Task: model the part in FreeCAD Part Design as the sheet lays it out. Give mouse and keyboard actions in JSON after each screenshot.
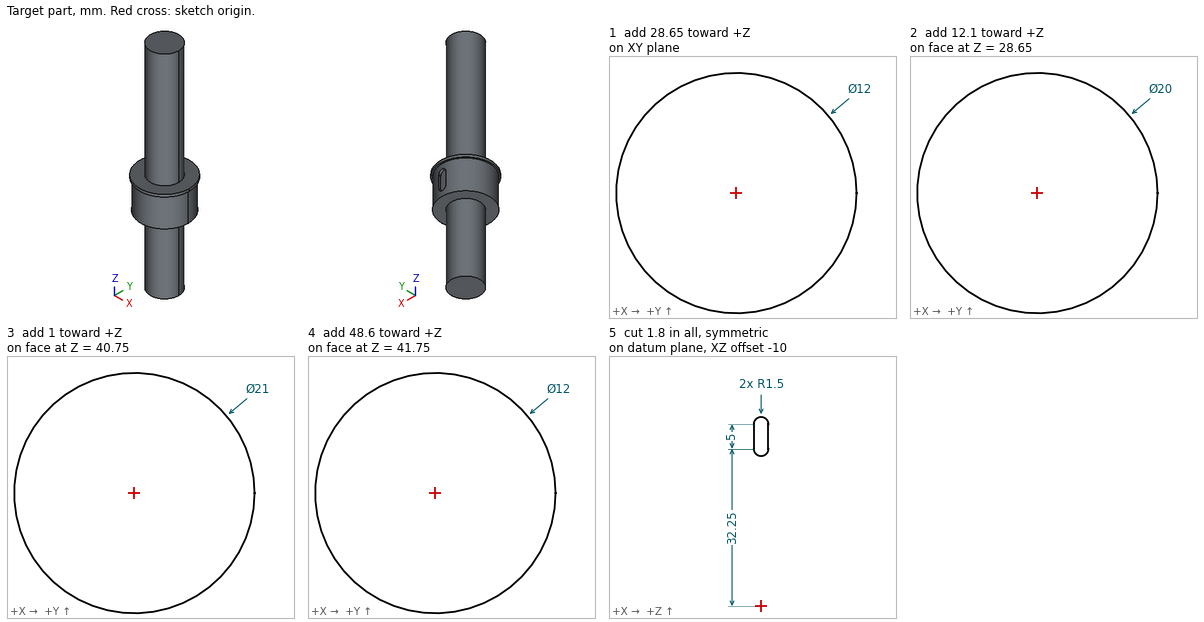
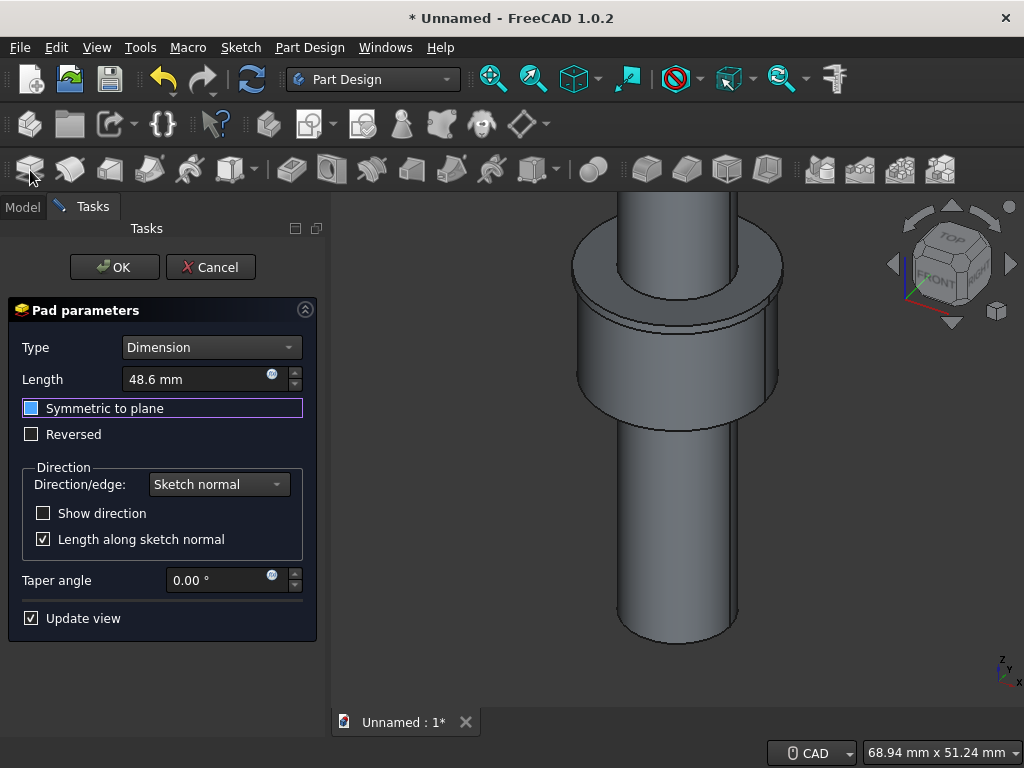
{"action": "left_click", "coordinate": [115, 267]}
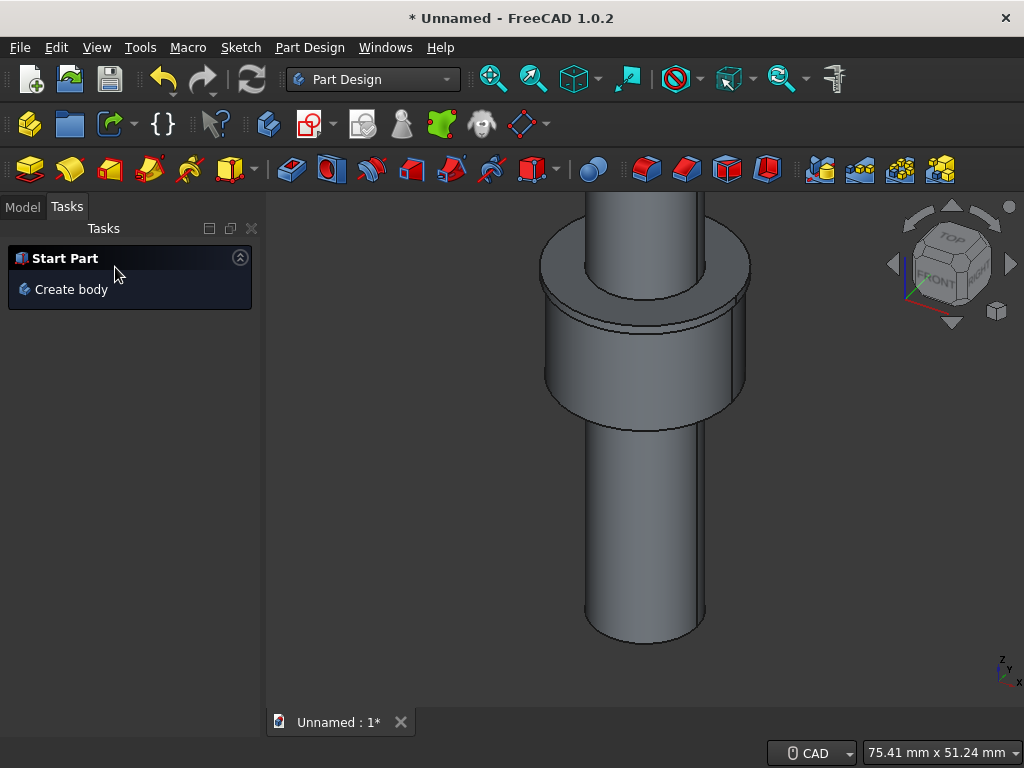
{"action": "left_click", "coordinate": [494, 80]}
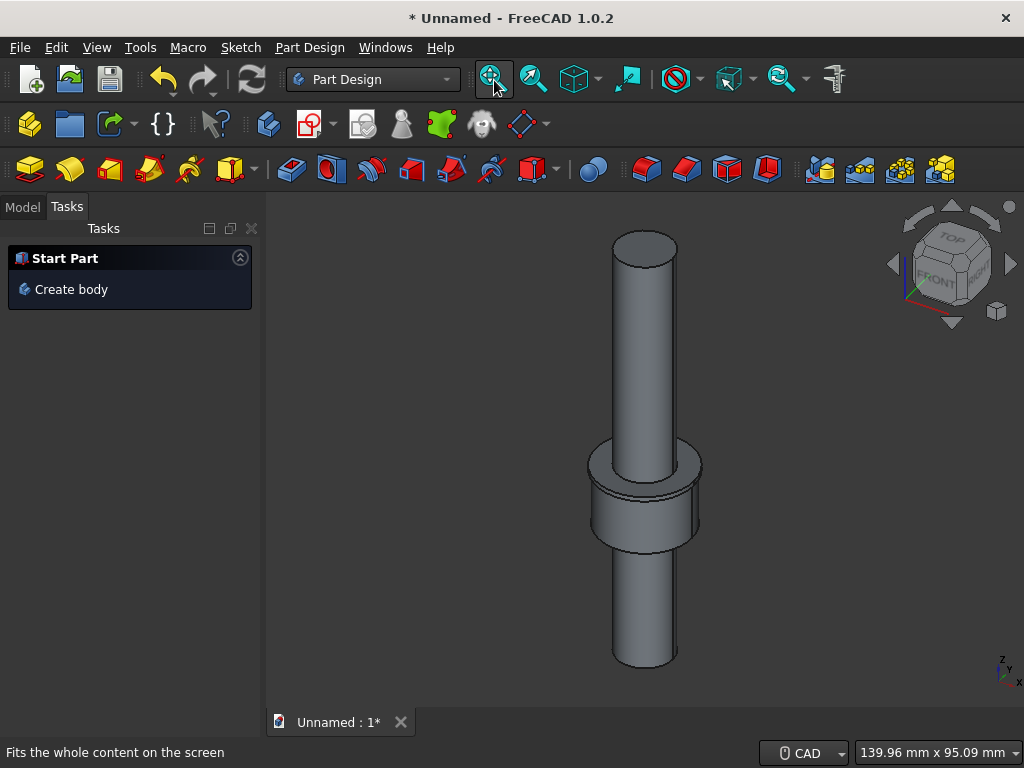
{"action": "left_click", "coordinate": [23, 206]}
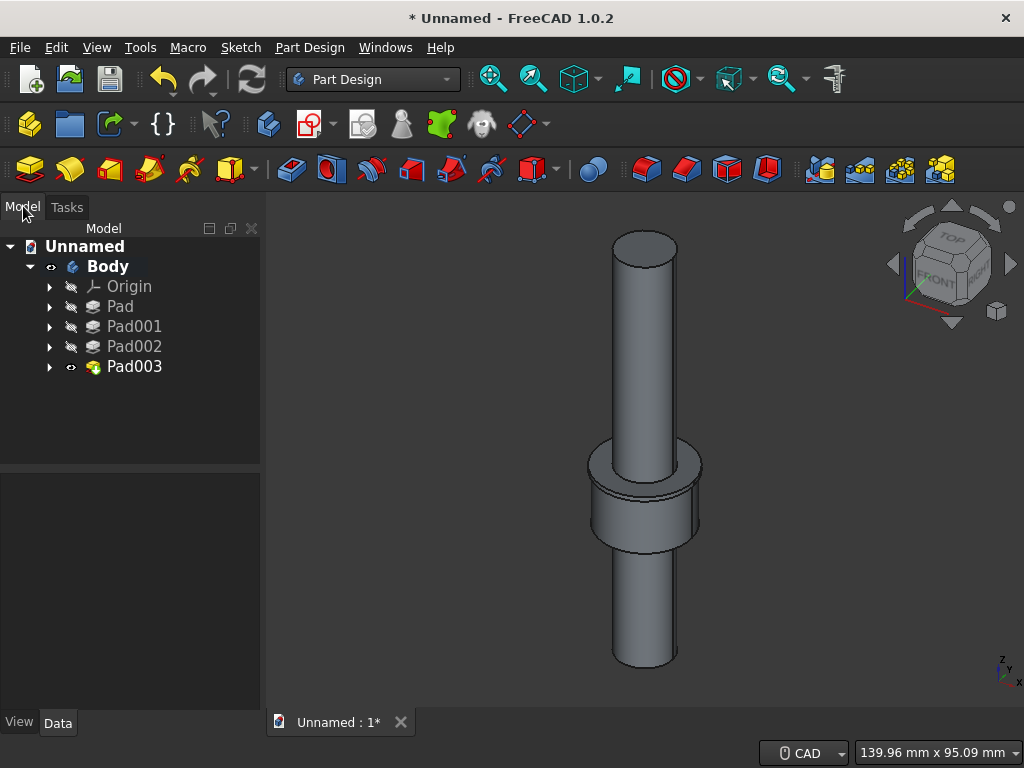
{"action": "left_click", "coordinate": [50, 287]}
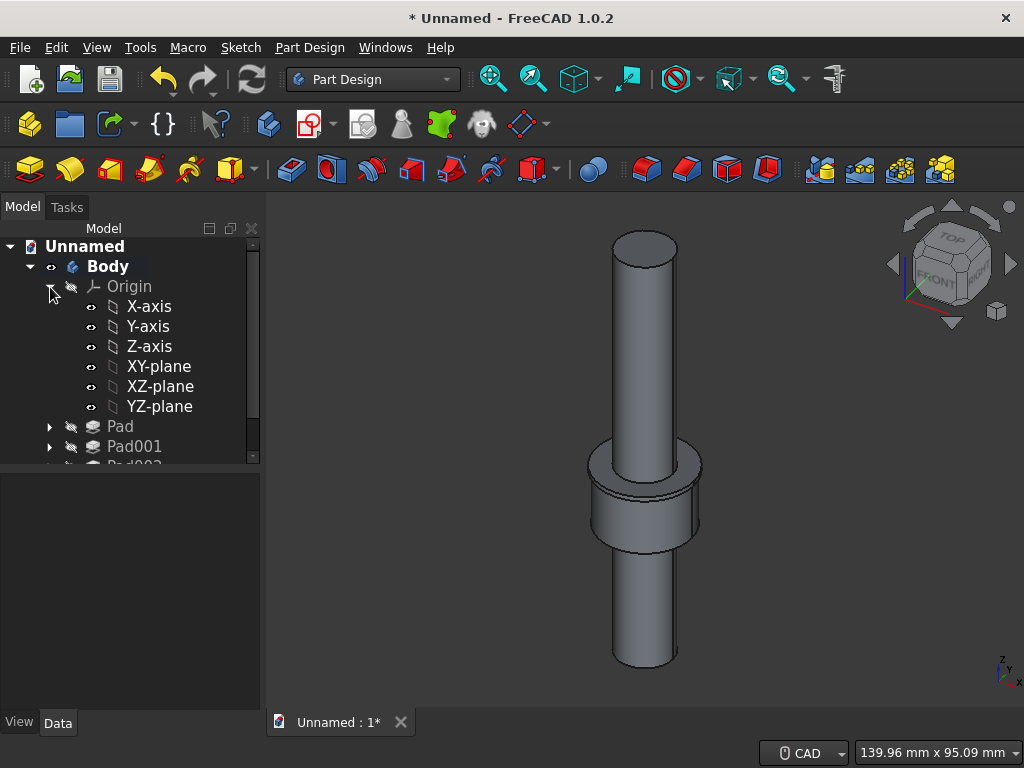
{"action": "left_click", "coordinate": [136, 387]}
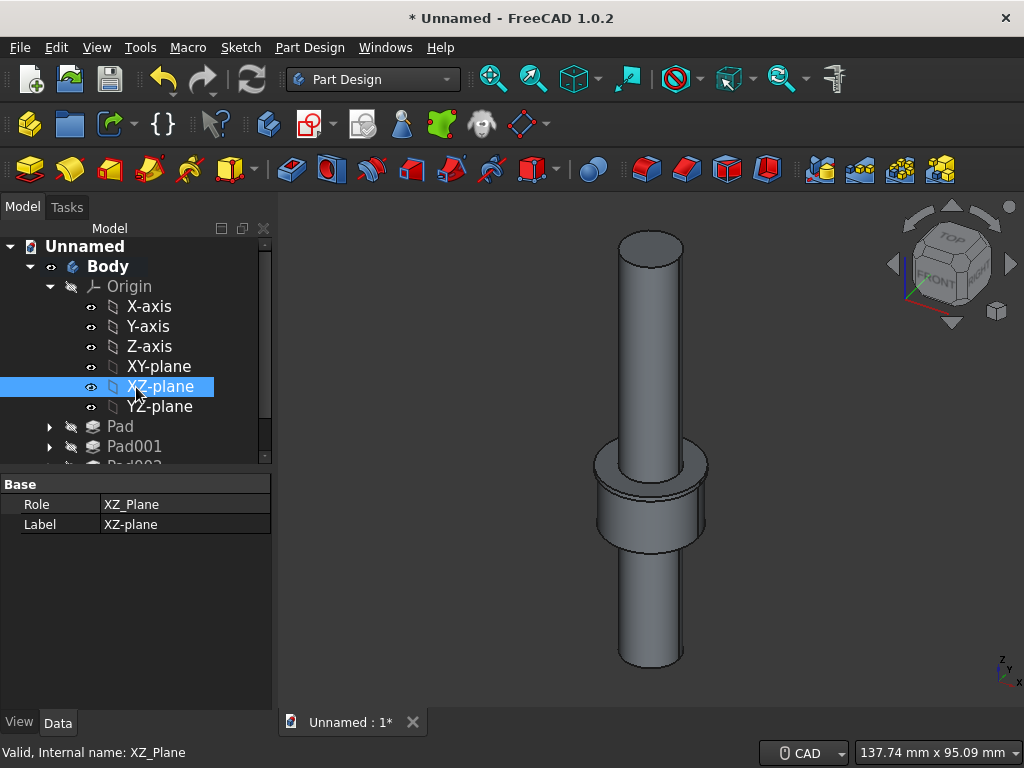
{"action": "left_click", "coordinate": [522, 124]}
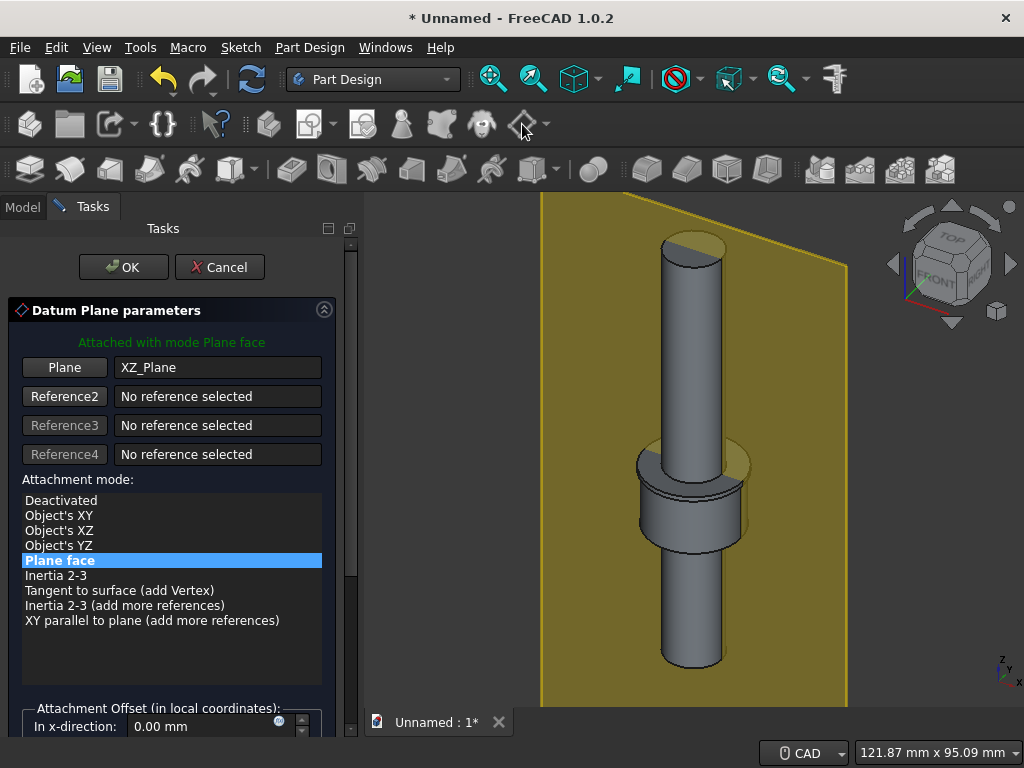
{"action": "scroll", "coordinate": [351, 487], "scroll_direction": "down", "scroll_amount": 3}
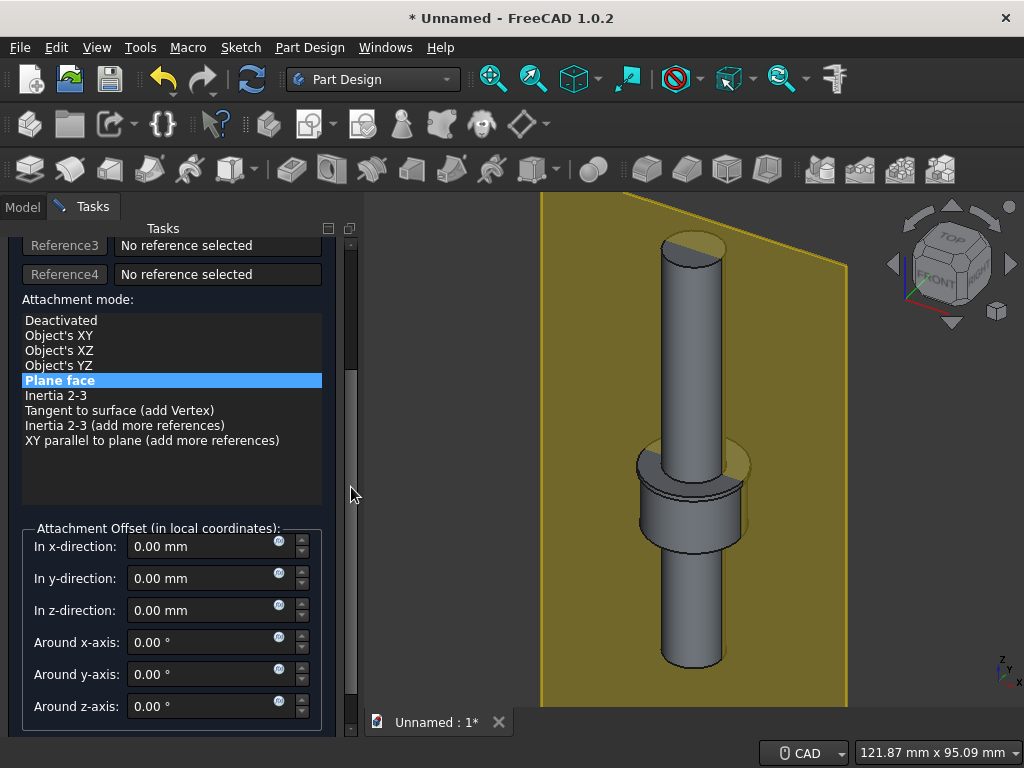
{"action": "triple_click", "coordinate": [210, 610]}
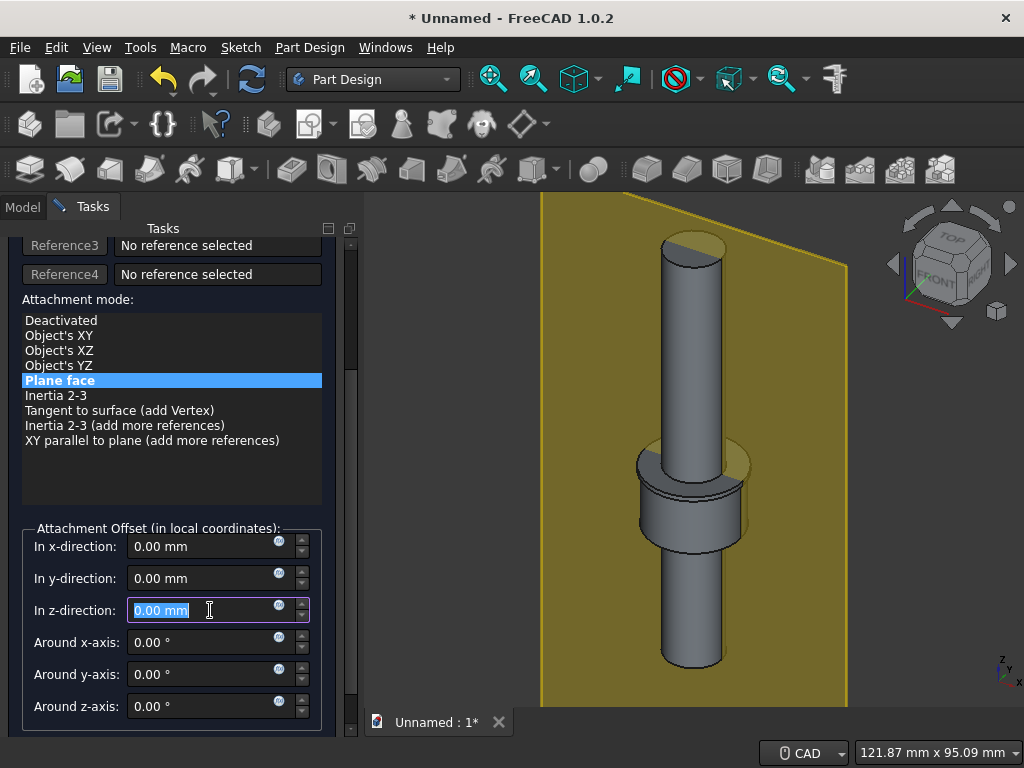
{"action": "type", "text": "-10"}
{"action": "key", "text": "Tab"}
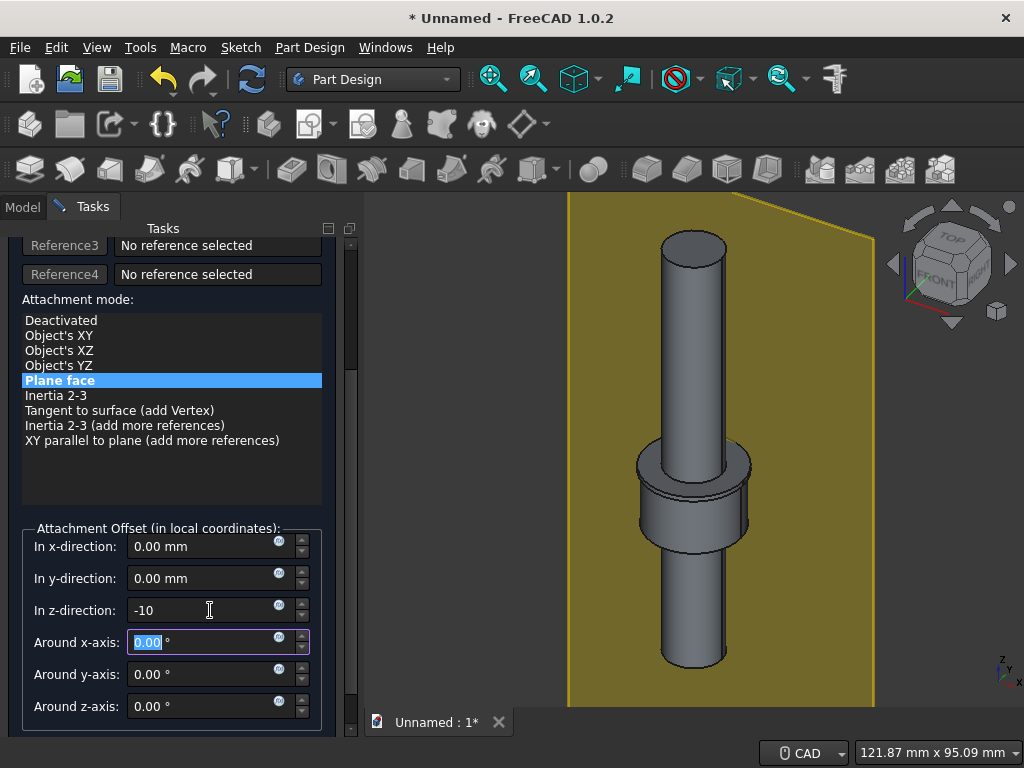
{"action": "scroll", "coordinate": [351, 487], "scroll_direction": "up", "scroll_amount": 4}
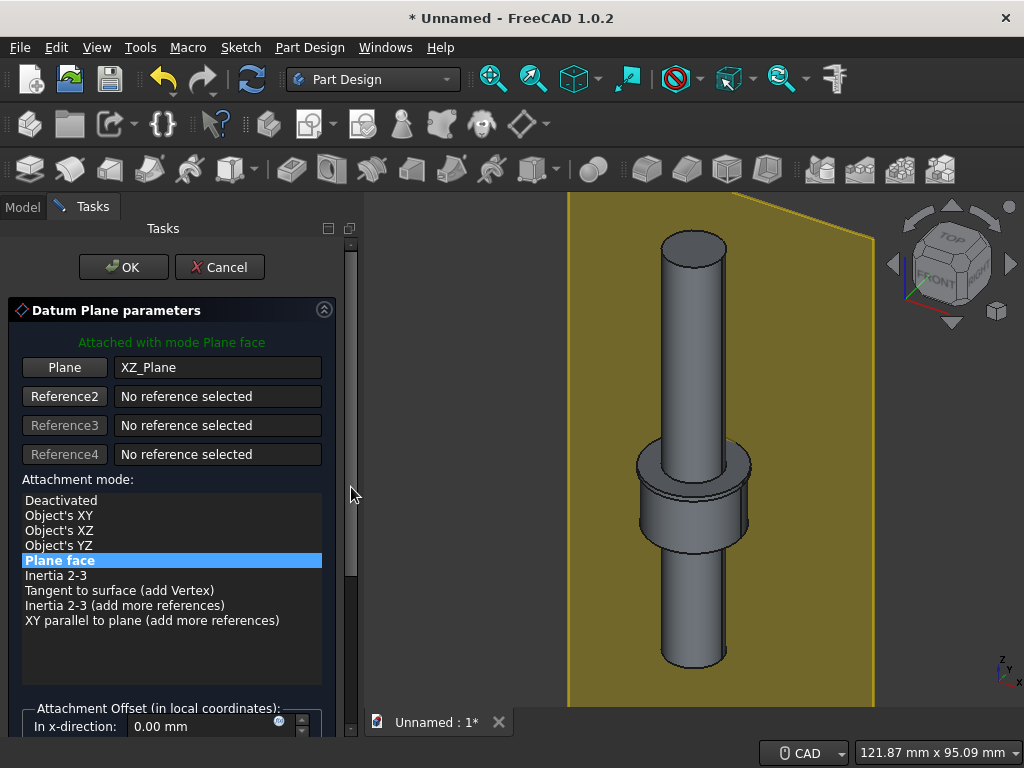
{"action": "left_click", "coordinate": [124, 267]}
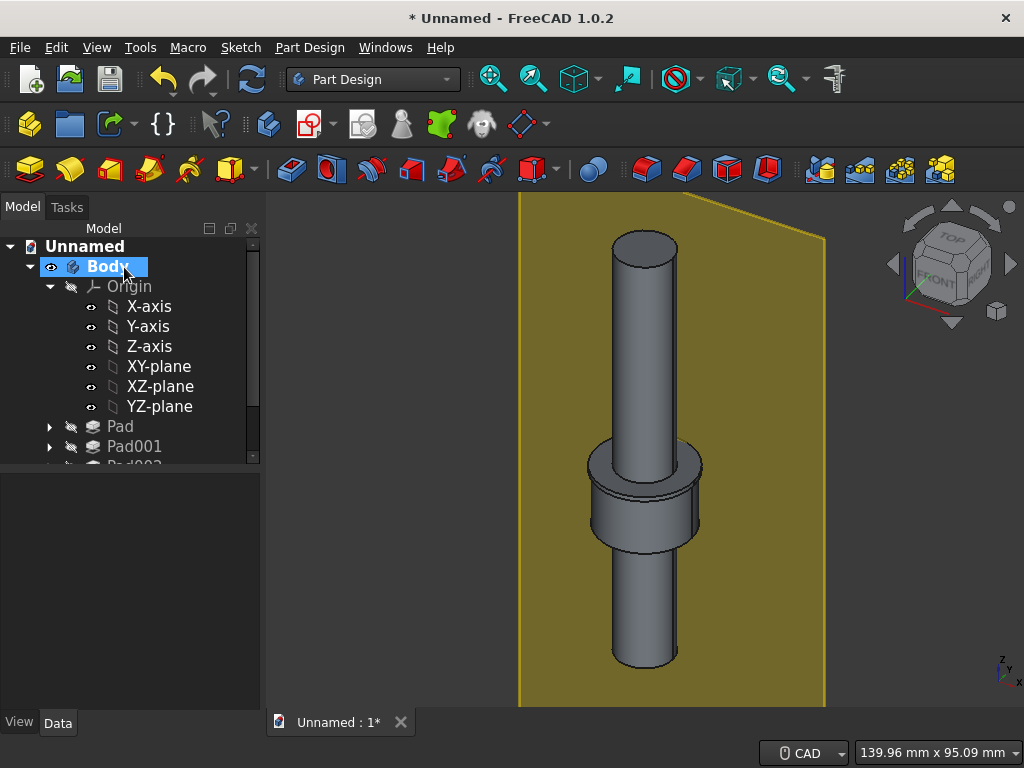
{"action": "scroll", "coordinate": [100, 342], "scroll_direction": "down", "scroll_amount": 3}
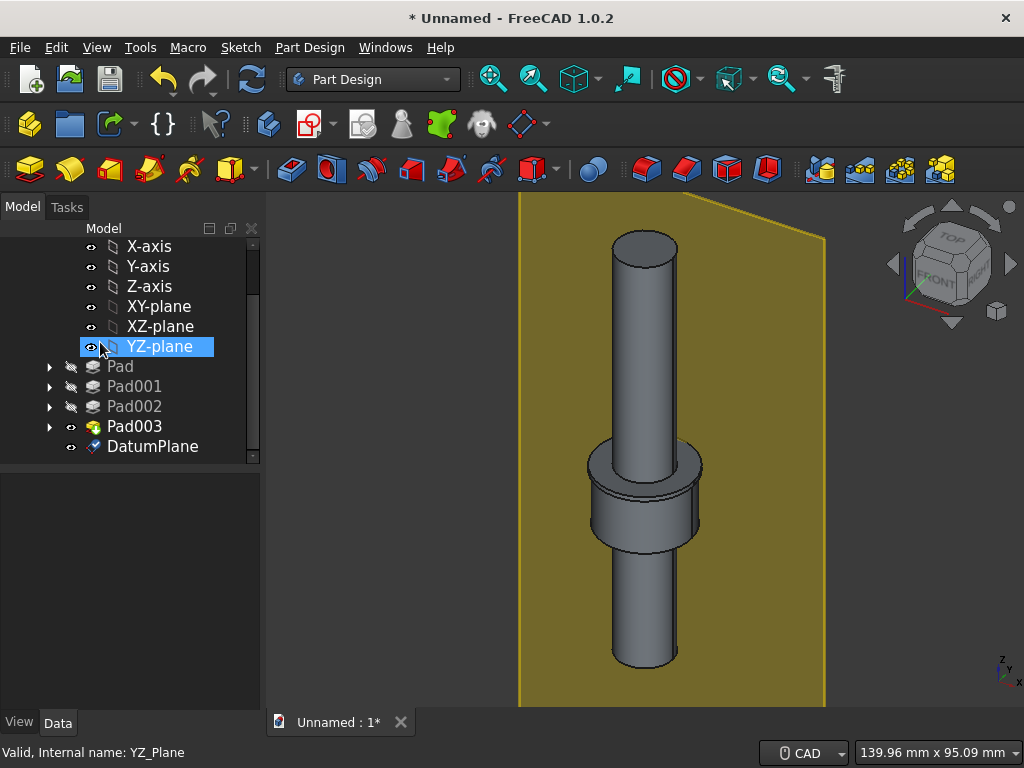
{"action": "left_click", "coordinate": [116, 447]}